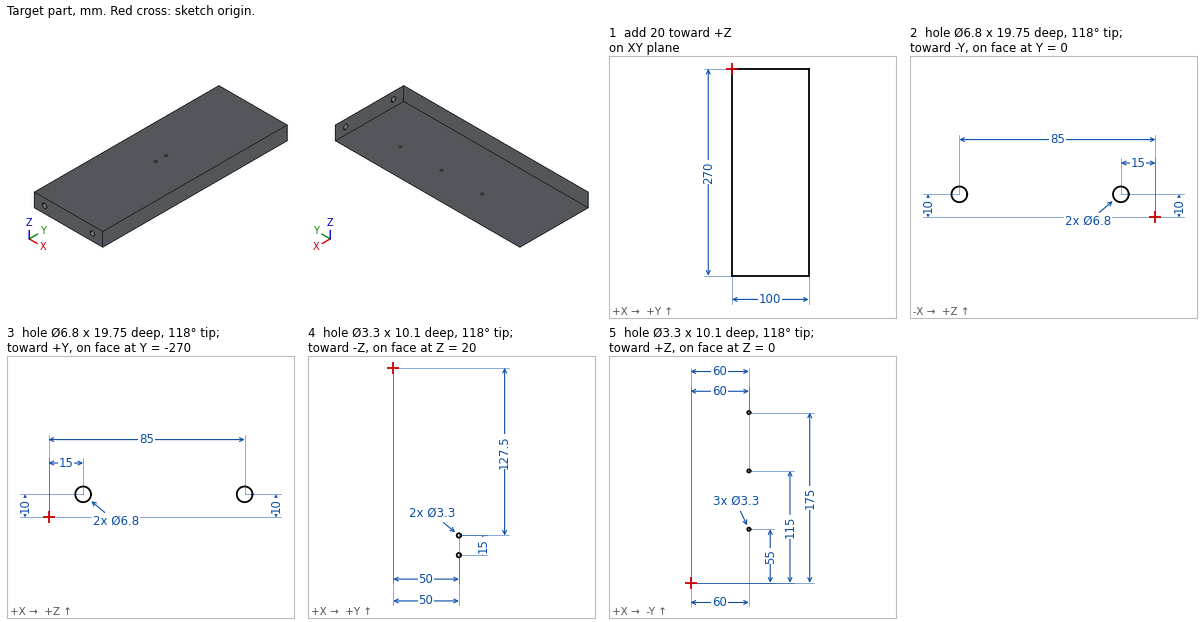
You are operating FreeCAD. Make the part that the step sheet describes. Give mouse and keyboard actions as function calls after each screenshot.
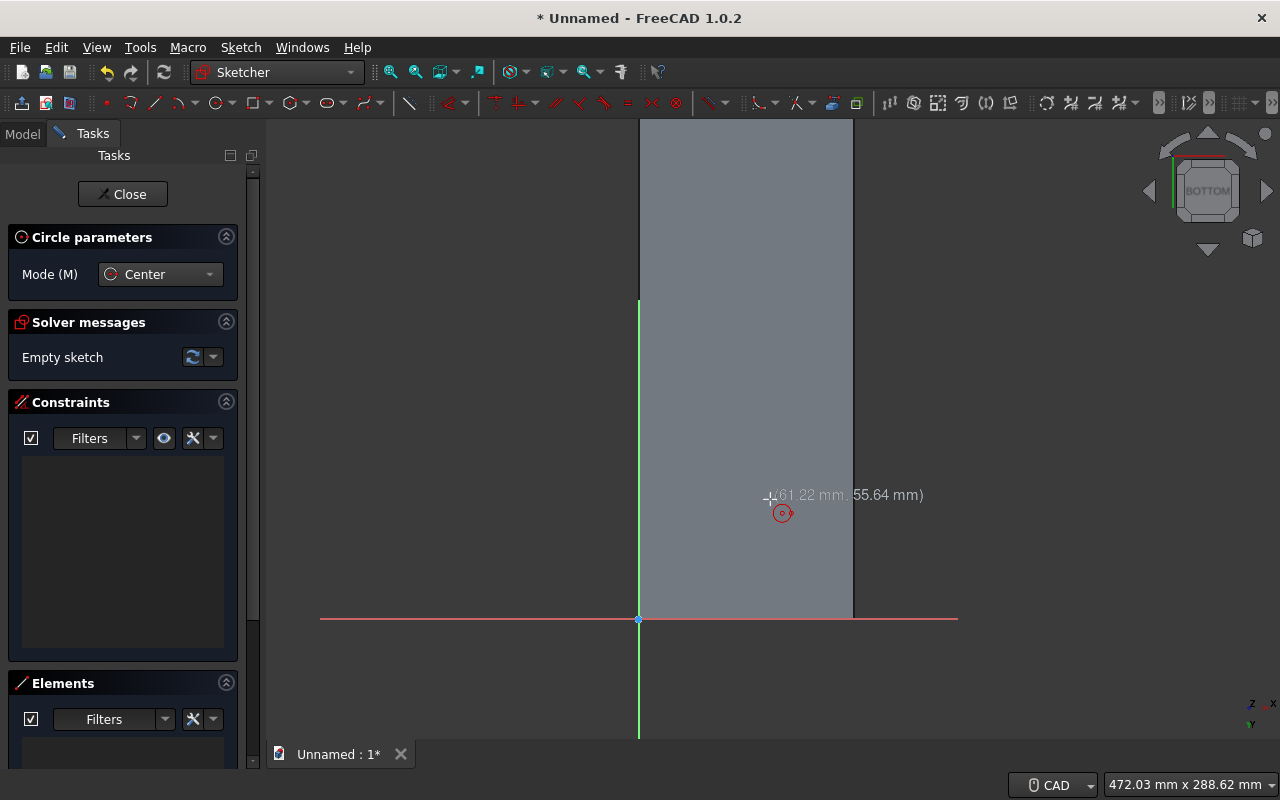
click(768, 501)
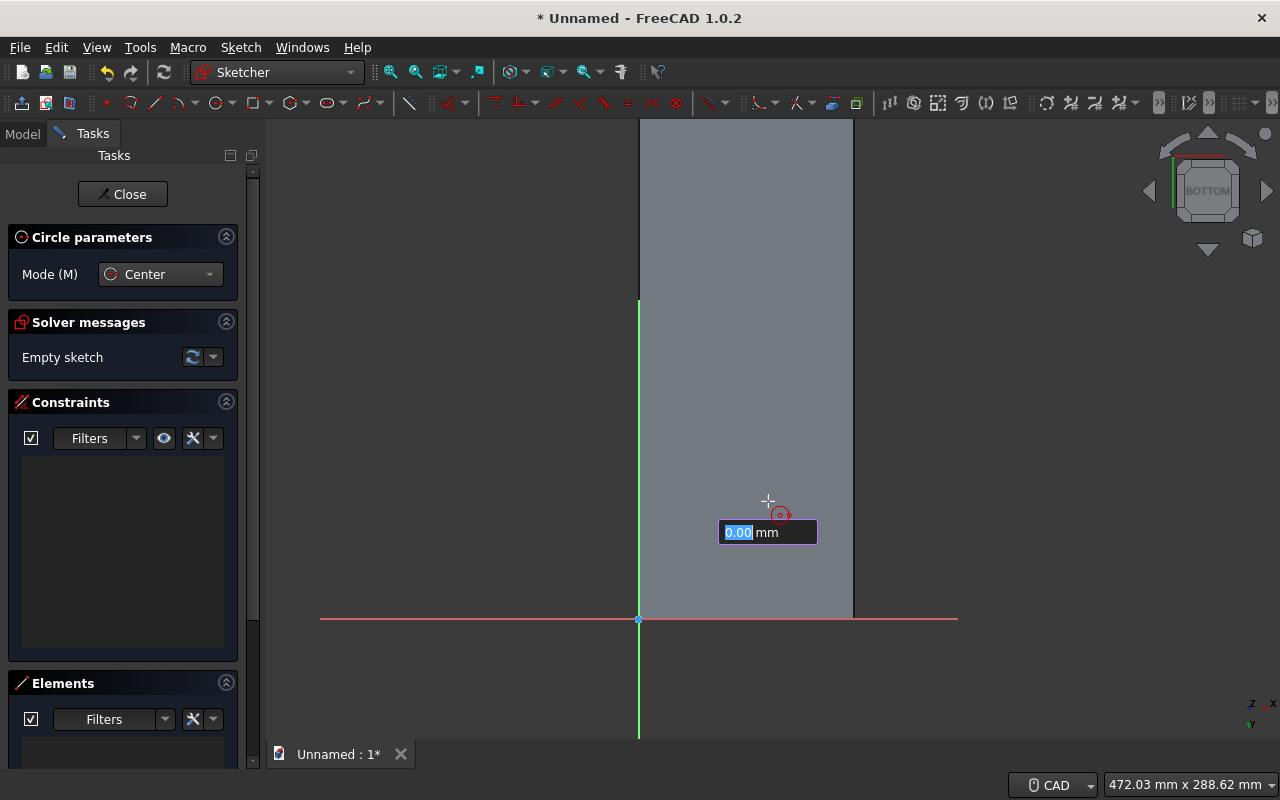
scroll(770, 499, up, 8)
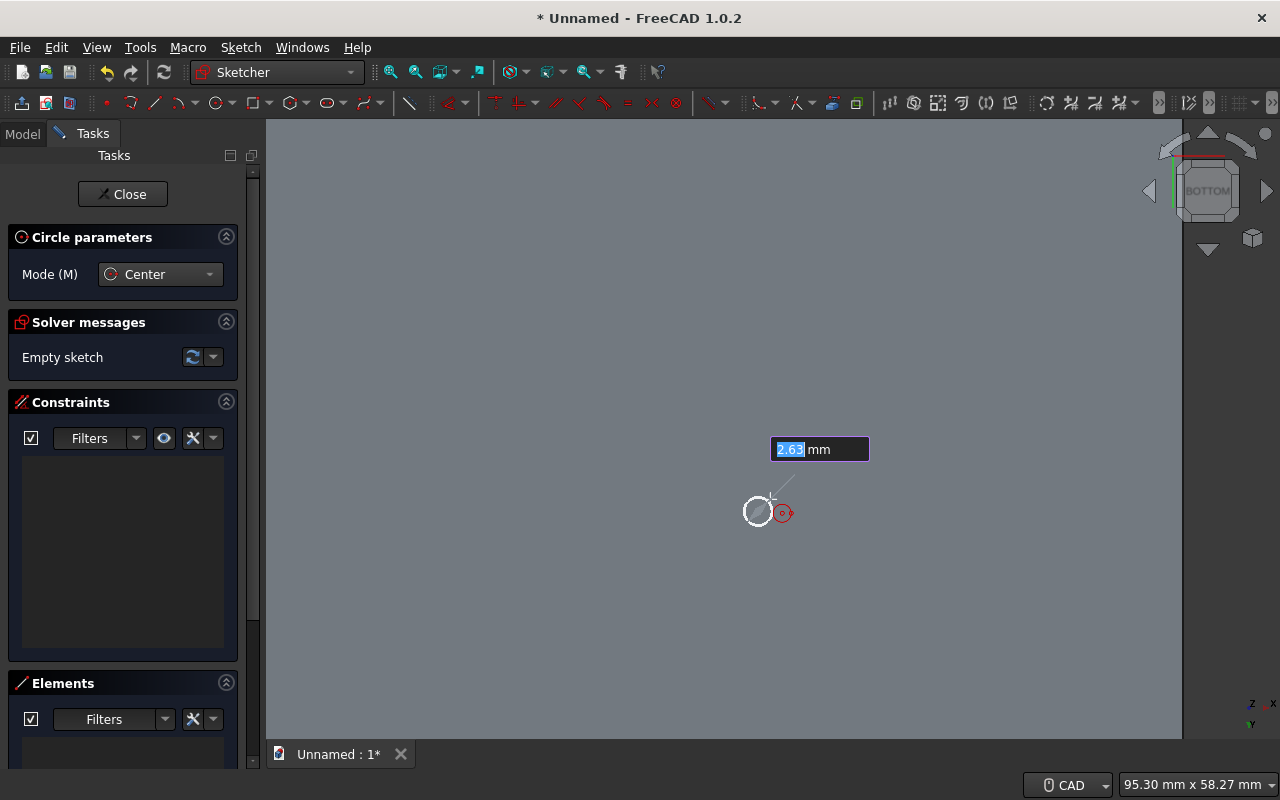
click(770, 494)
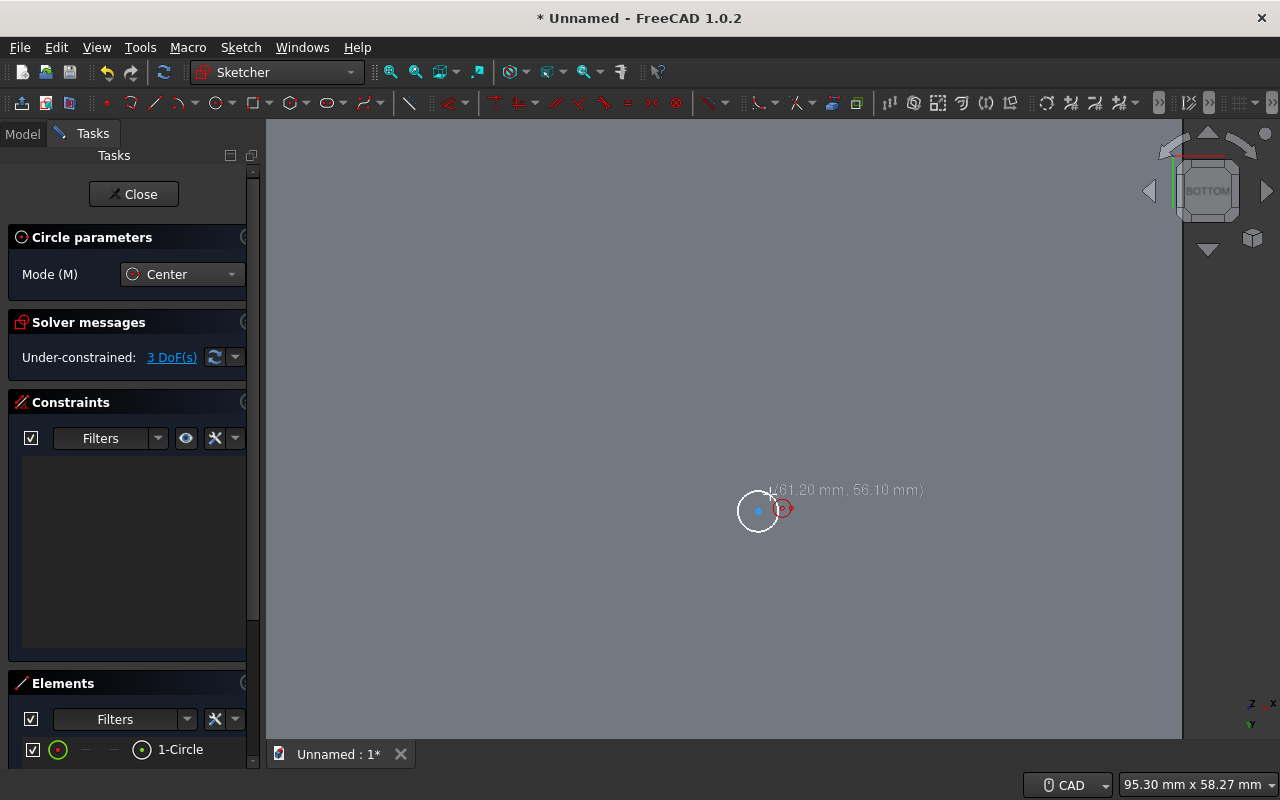
scroll(770, 499, down, 8)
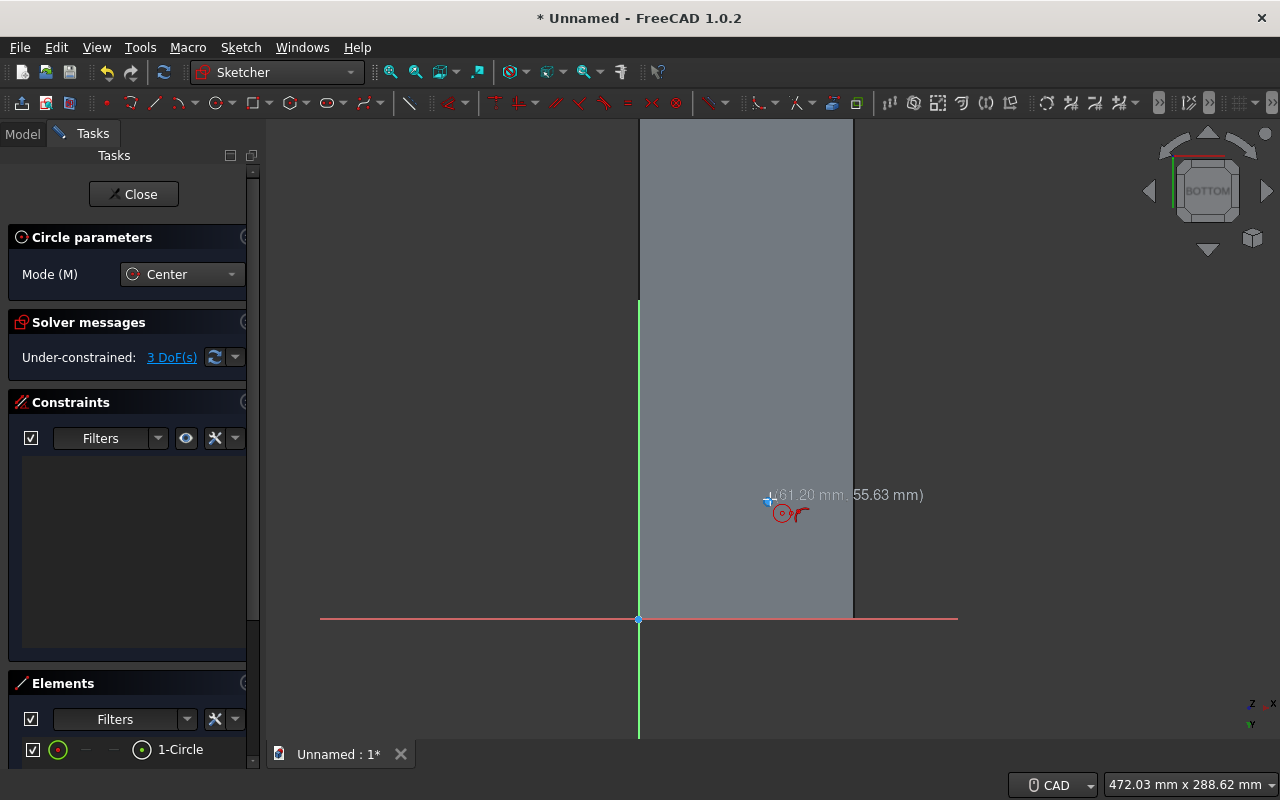
scroll(768, 372, up, 10)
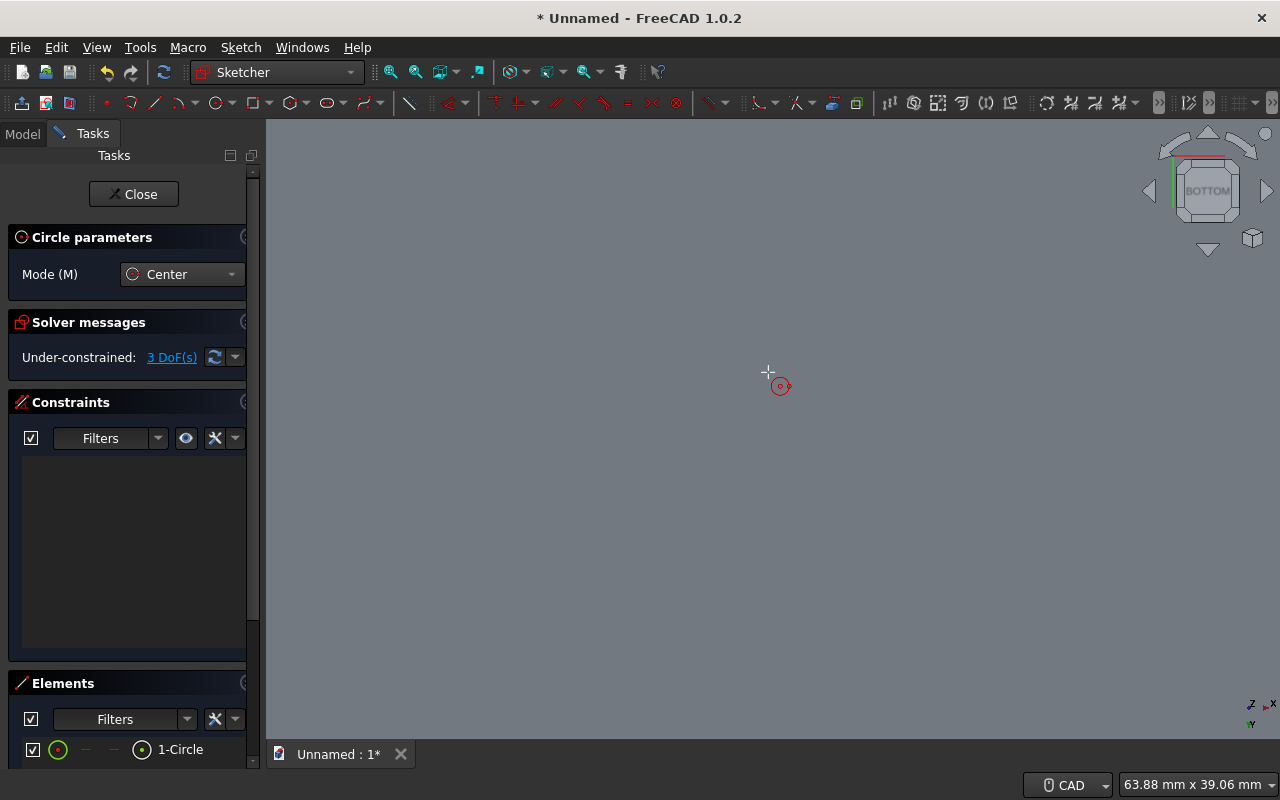
scroll(768, 372, down, 10)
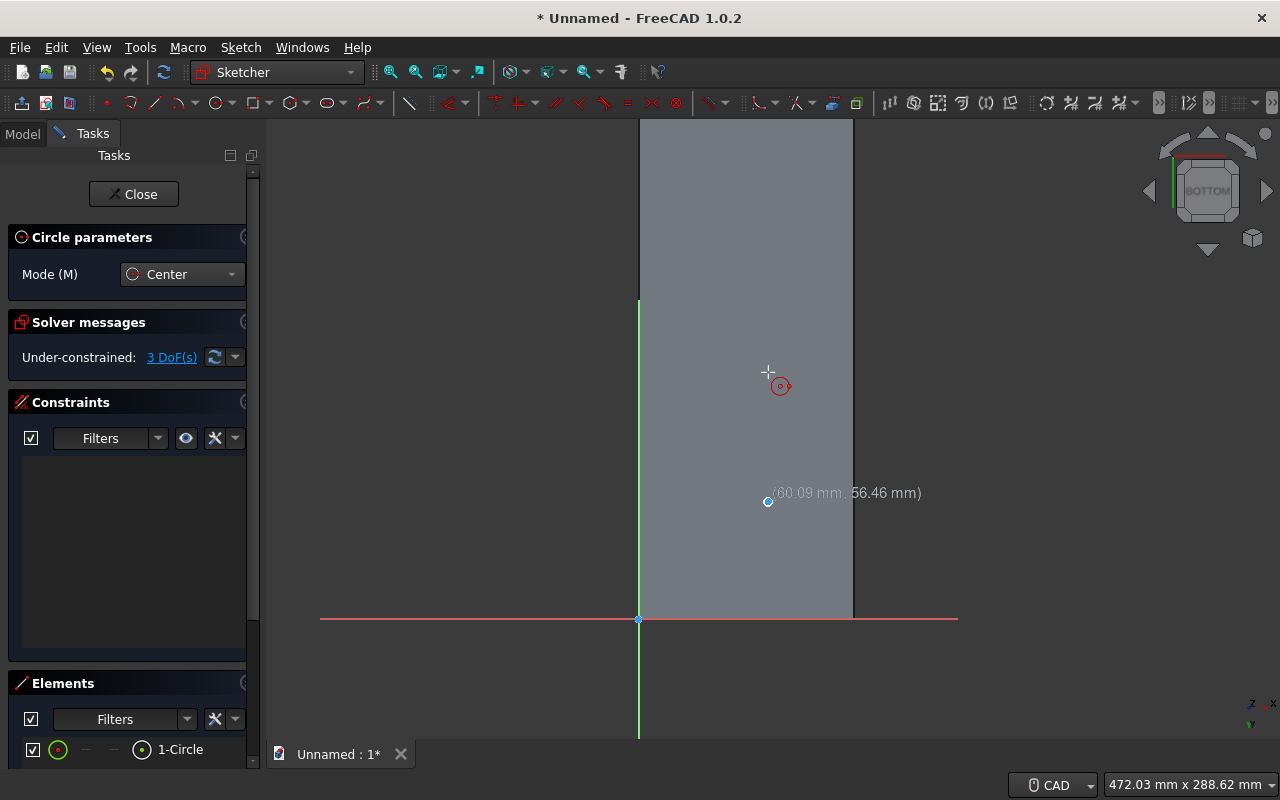
click(768, 372)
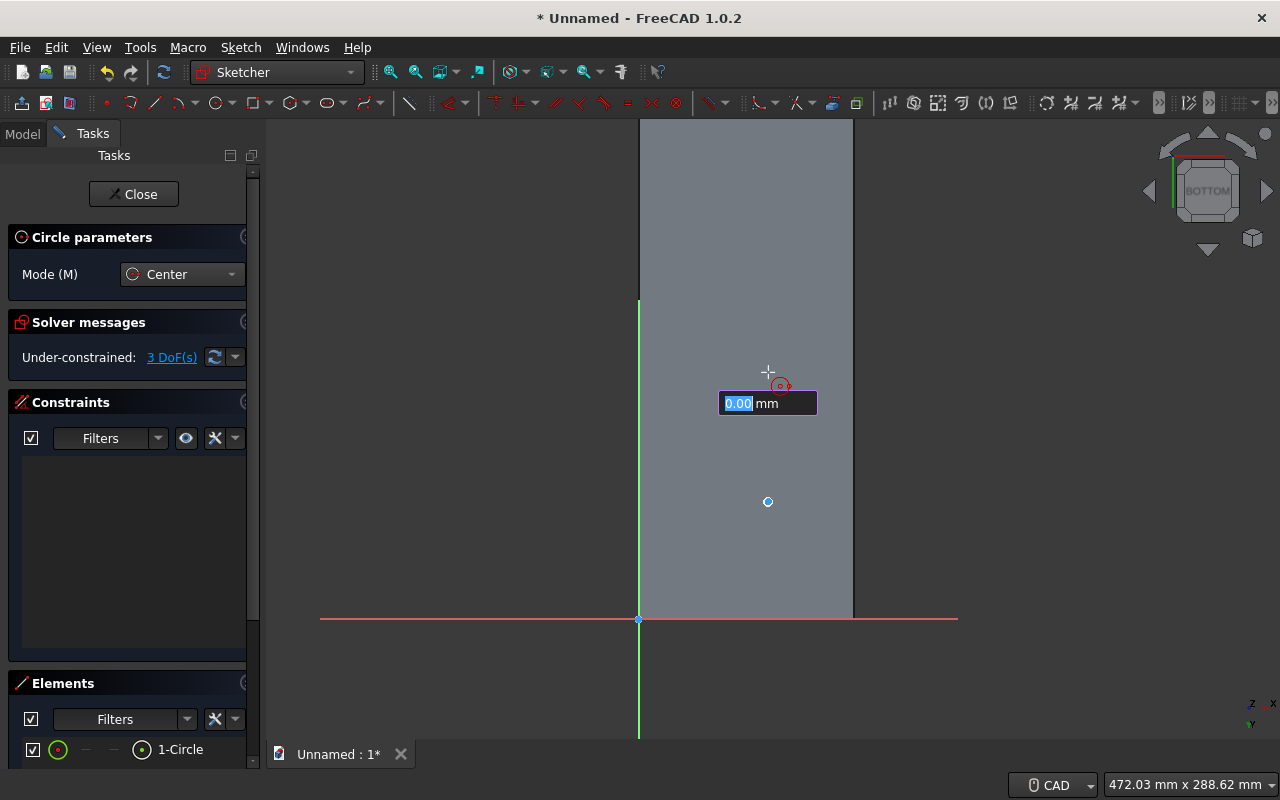
scroll(770, 370, up, 8)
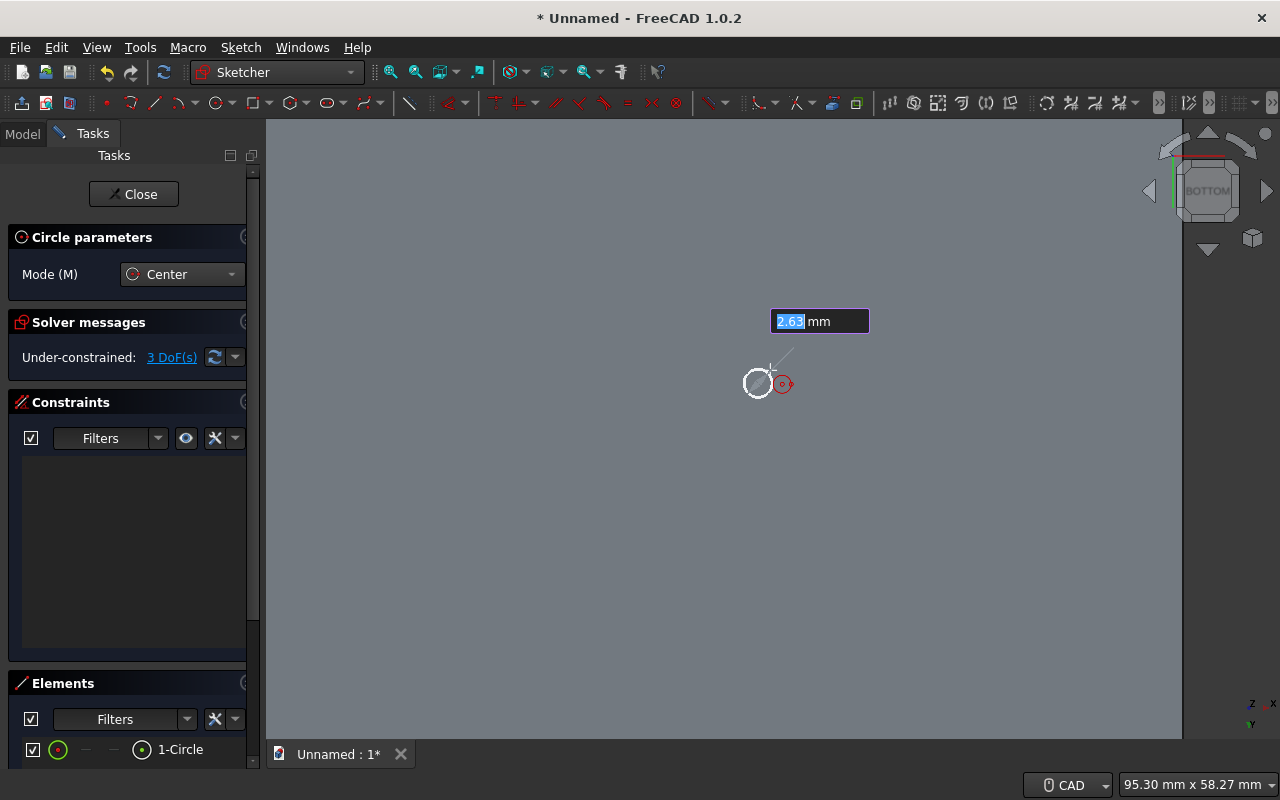
click(770, 367)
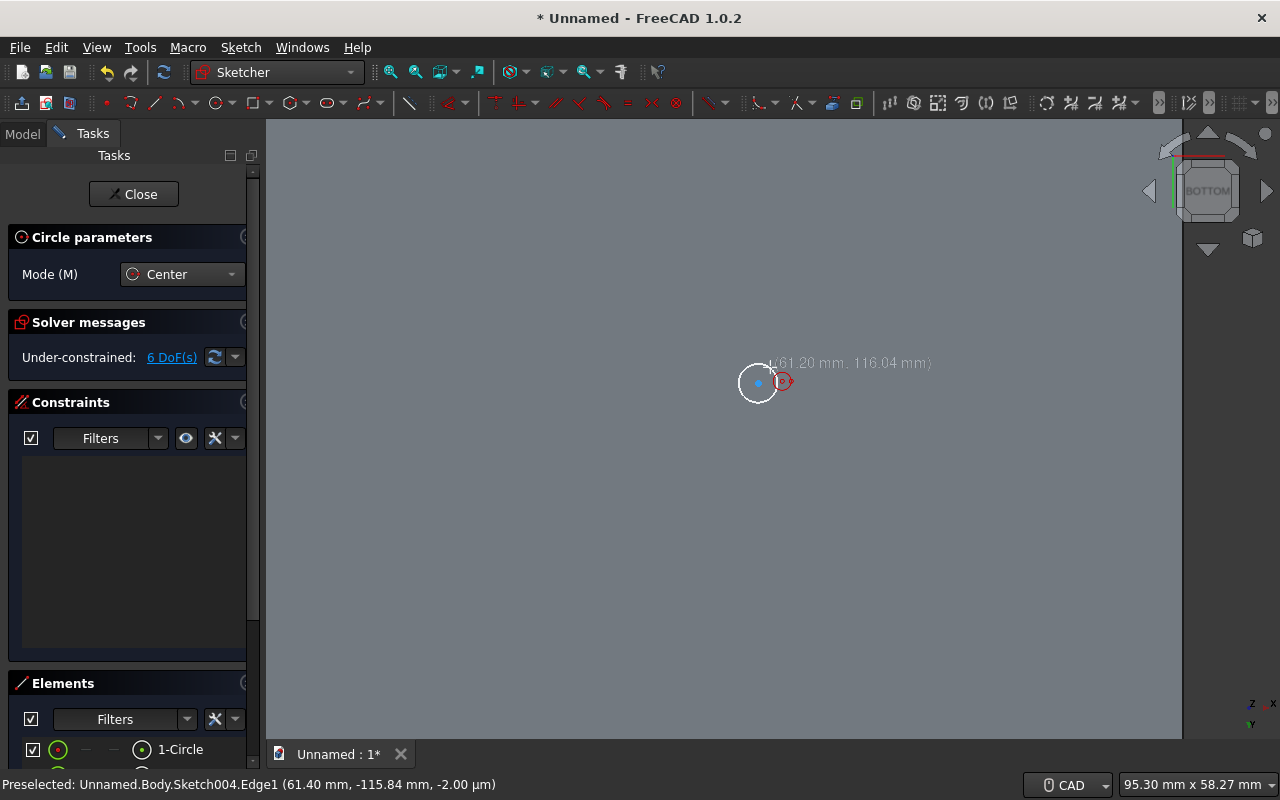
scroll(770, 370, down, 8)